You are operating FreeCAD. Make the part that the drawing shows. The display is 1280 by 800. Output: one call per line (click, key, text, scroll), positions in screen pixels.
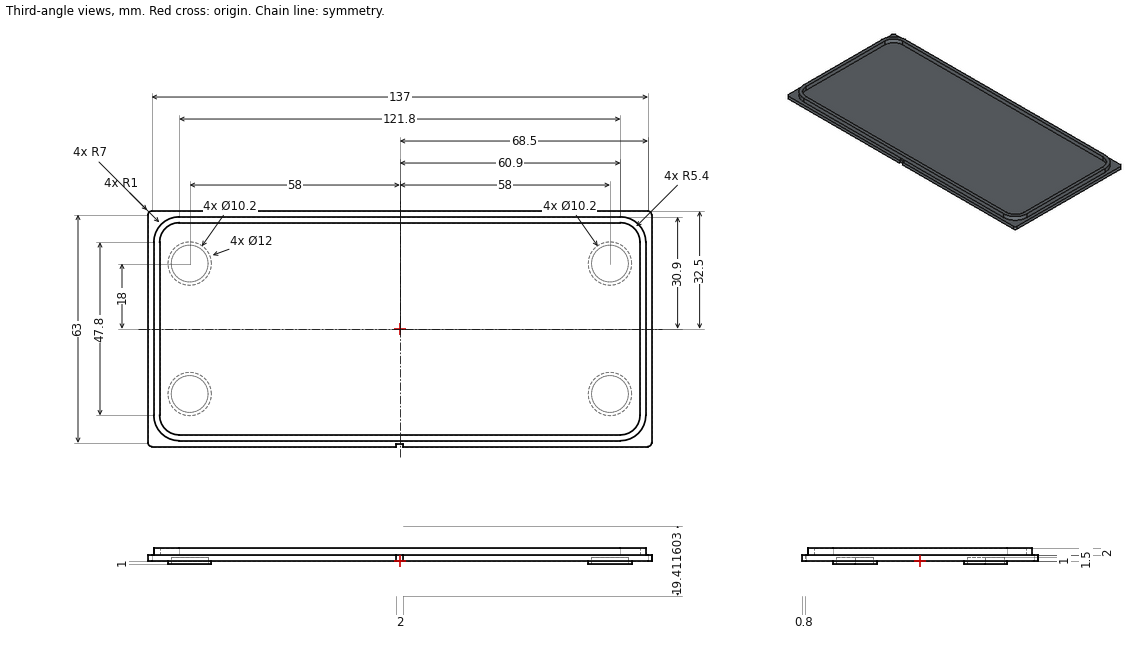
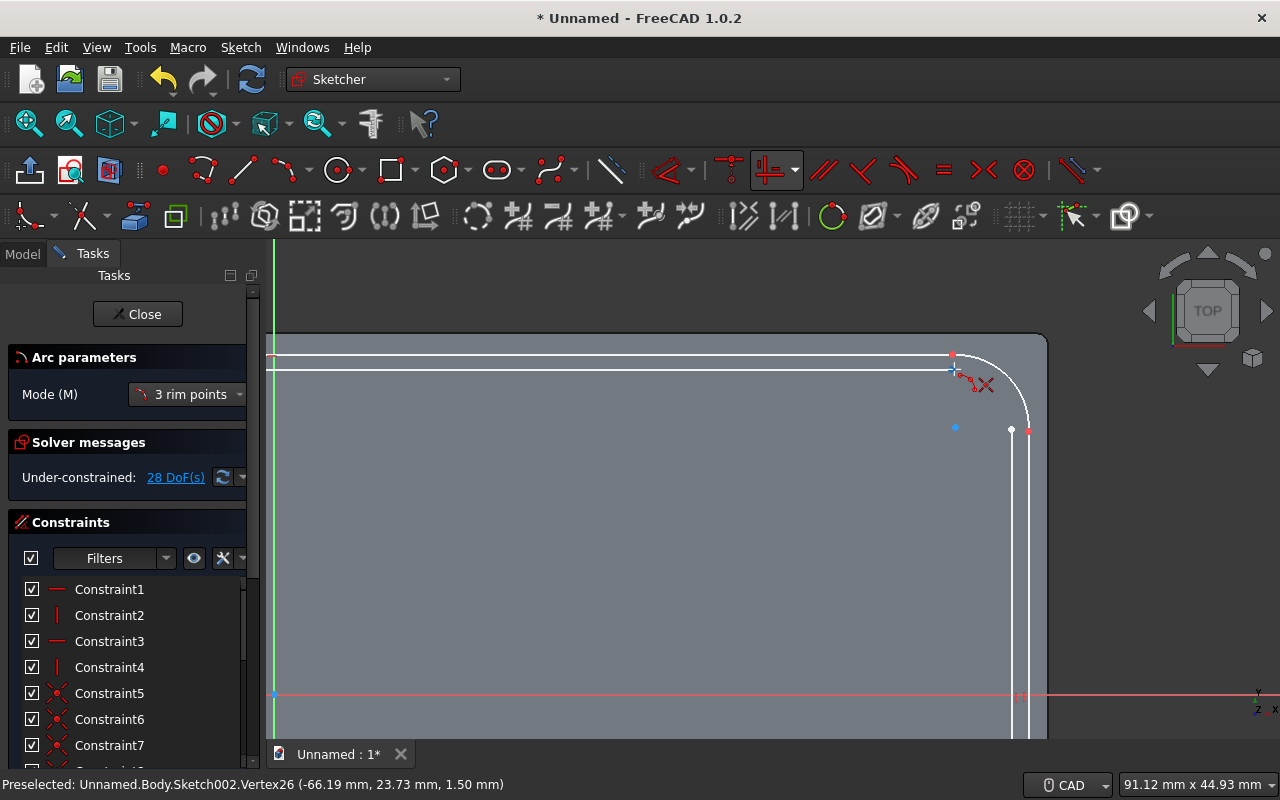
click(952, 370)
click(1012, 430)
click(995, 387)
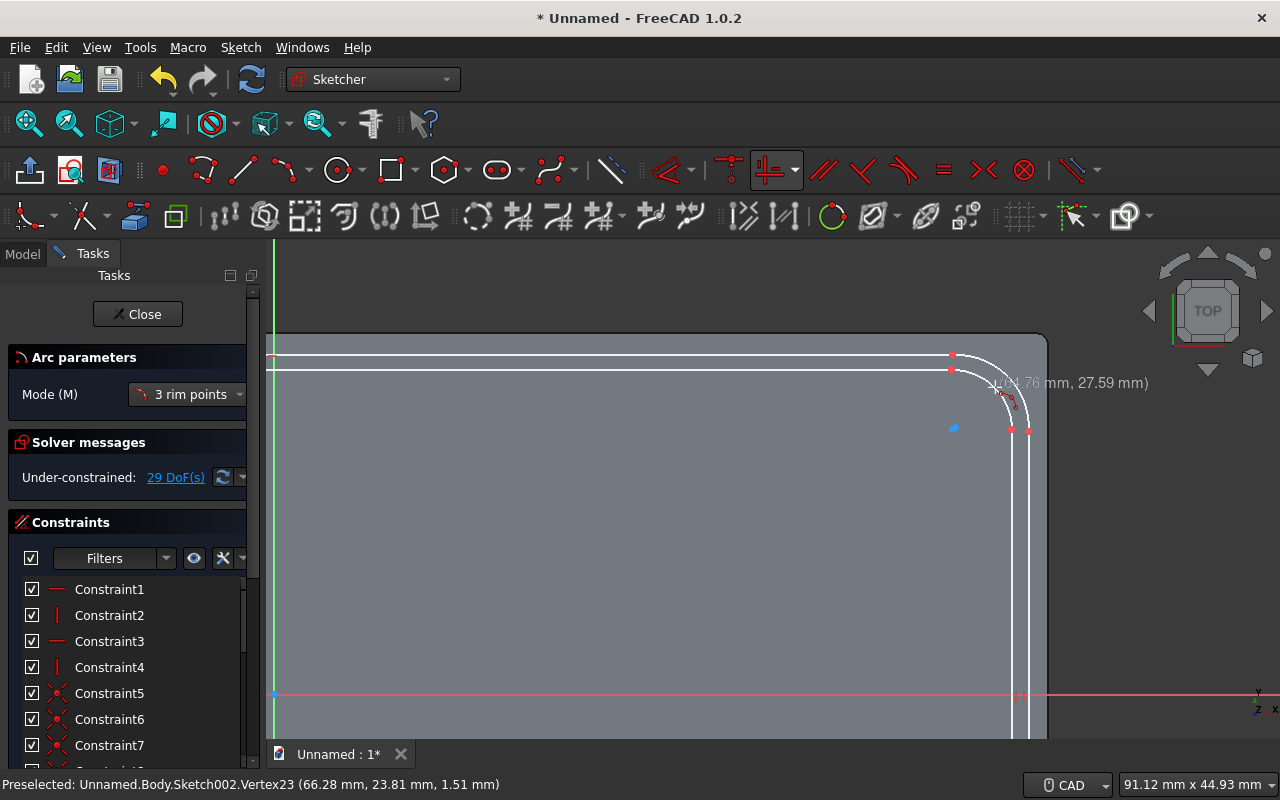
scroll(955, 369, down, 5)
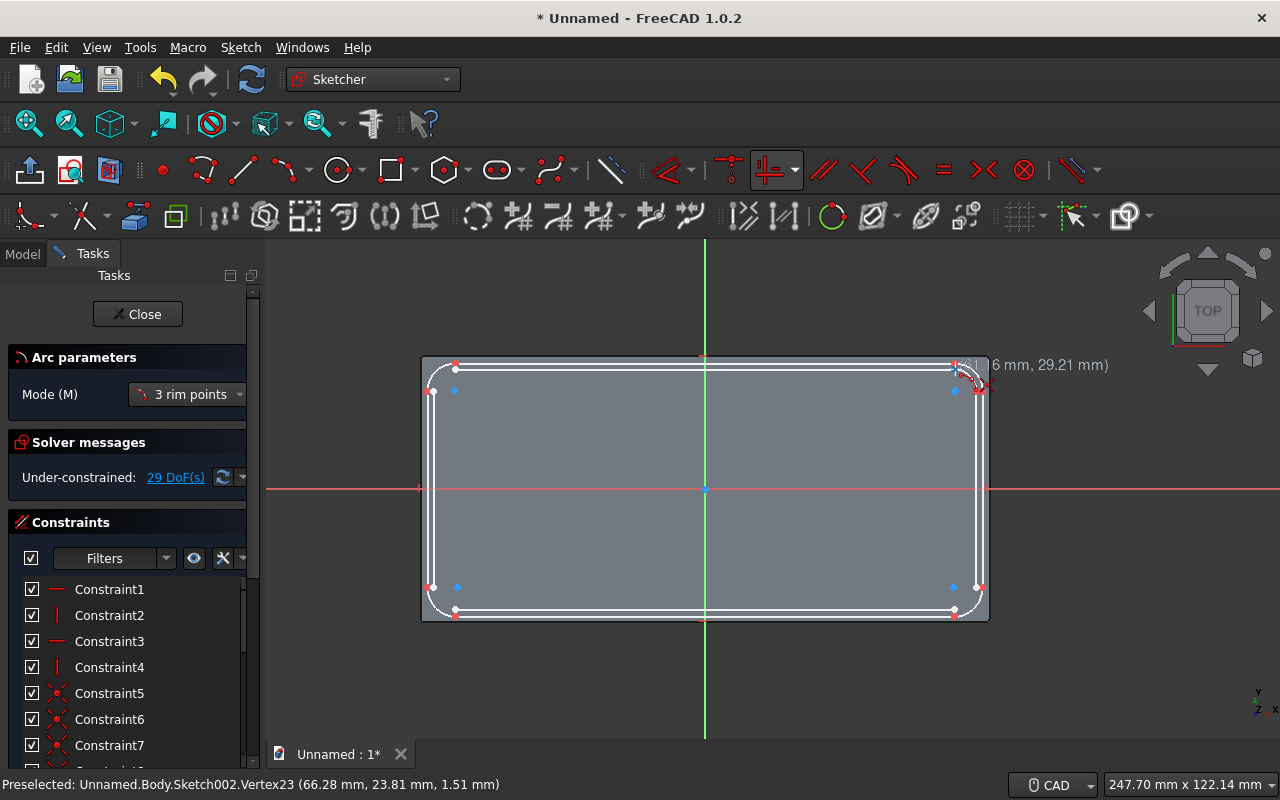
scroll(976, 587, up, 5)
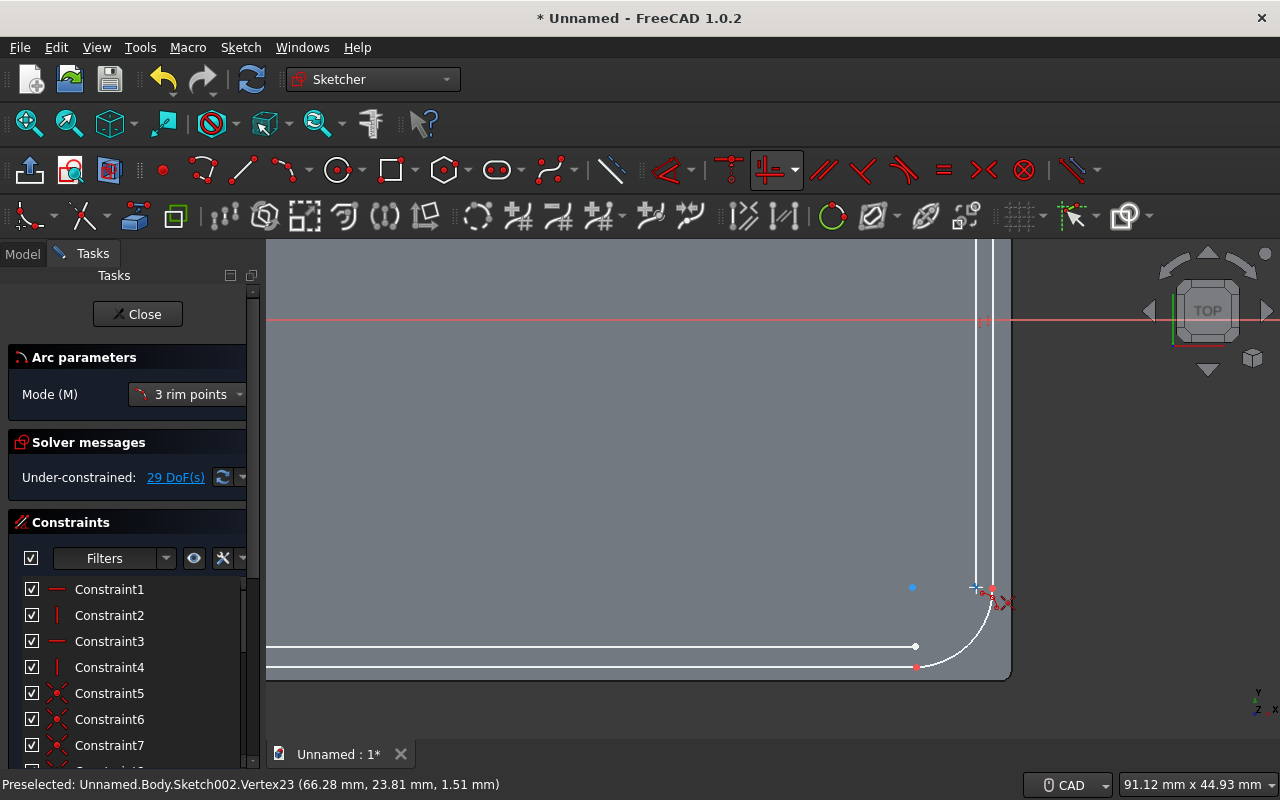
click(976, 587)
click(916, 647)
click(958, 628)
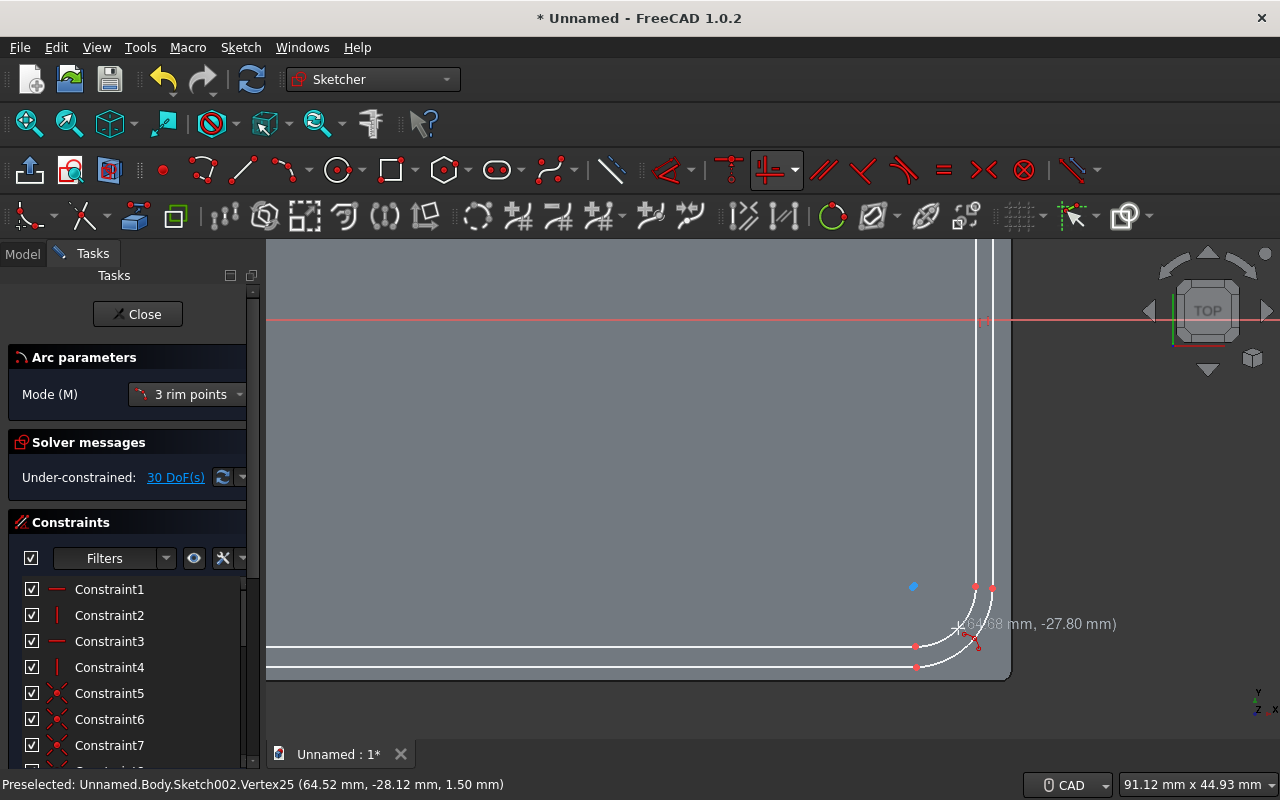
scroll(976, 588, down, 5)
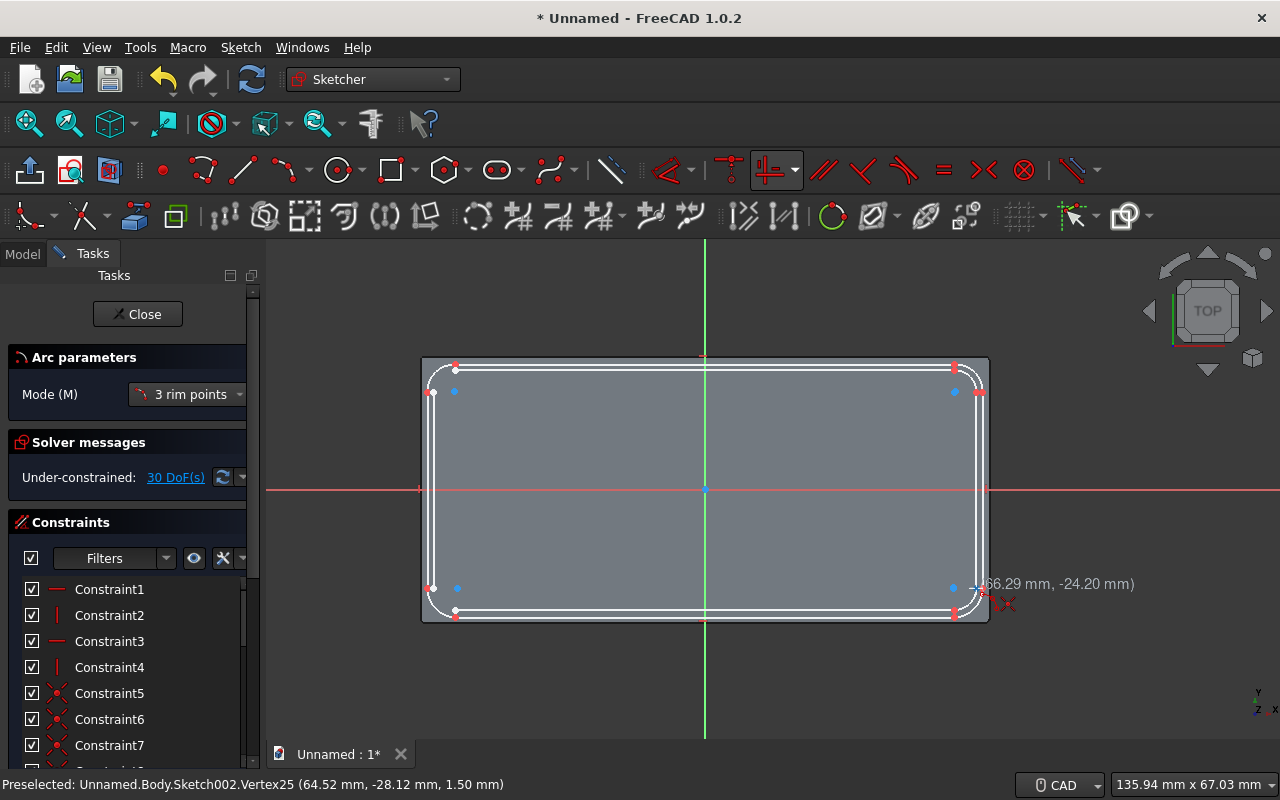
scroll(456, 610, up, 5)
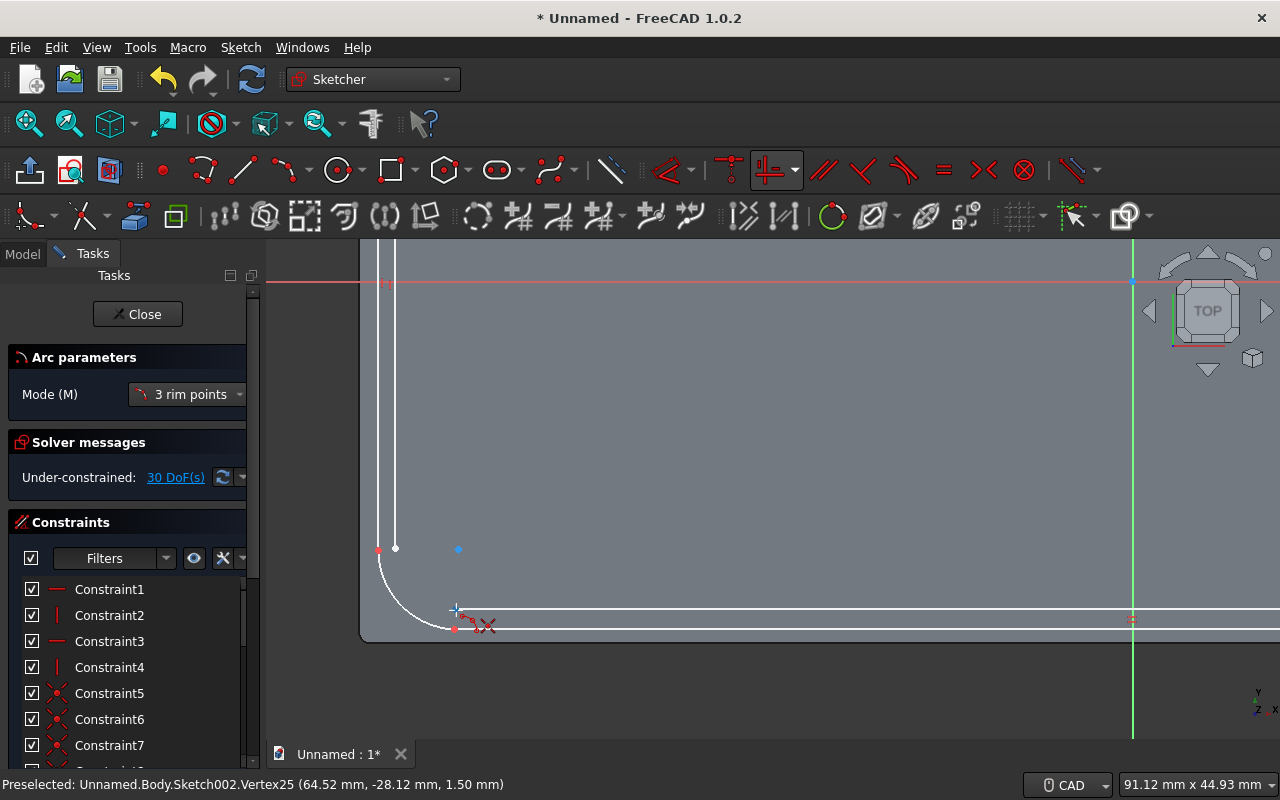
click(455, 609)
click(395, 549)
click(413, 590)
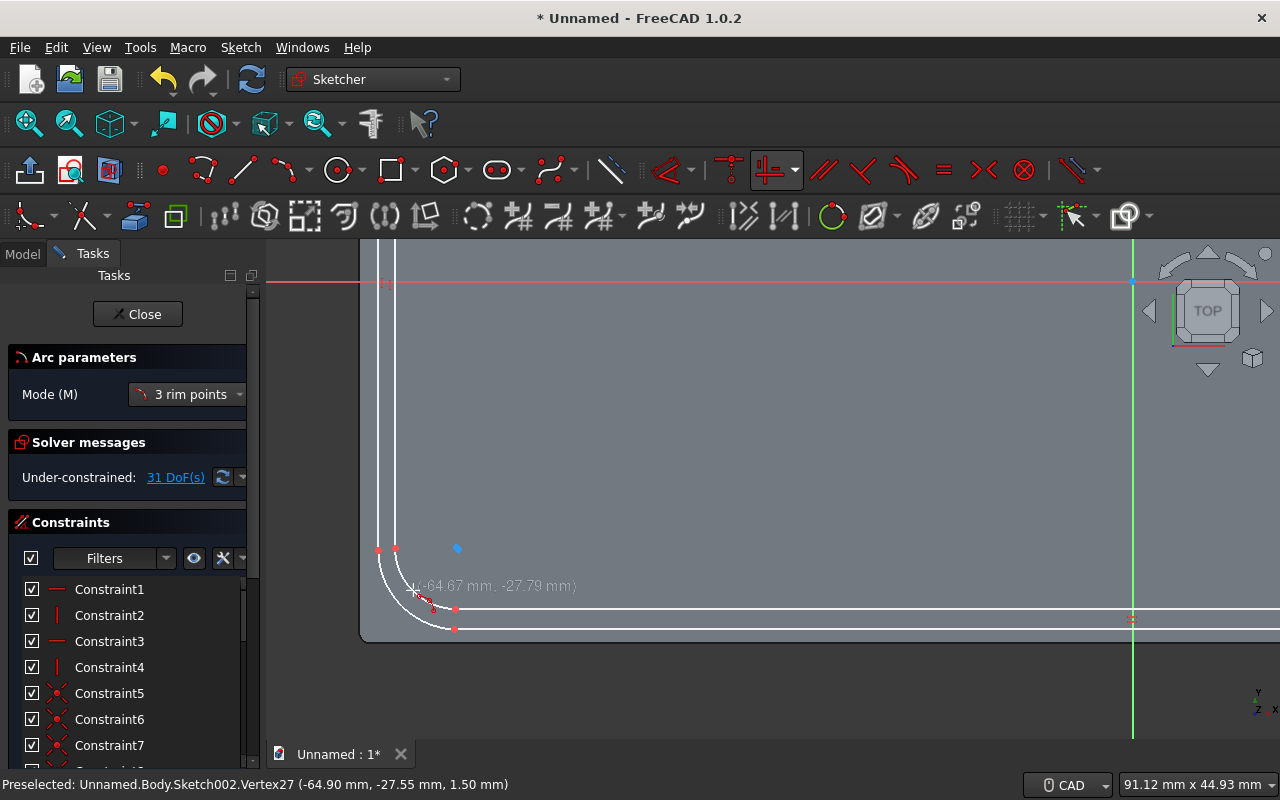
scroll(455, 610, down, 5)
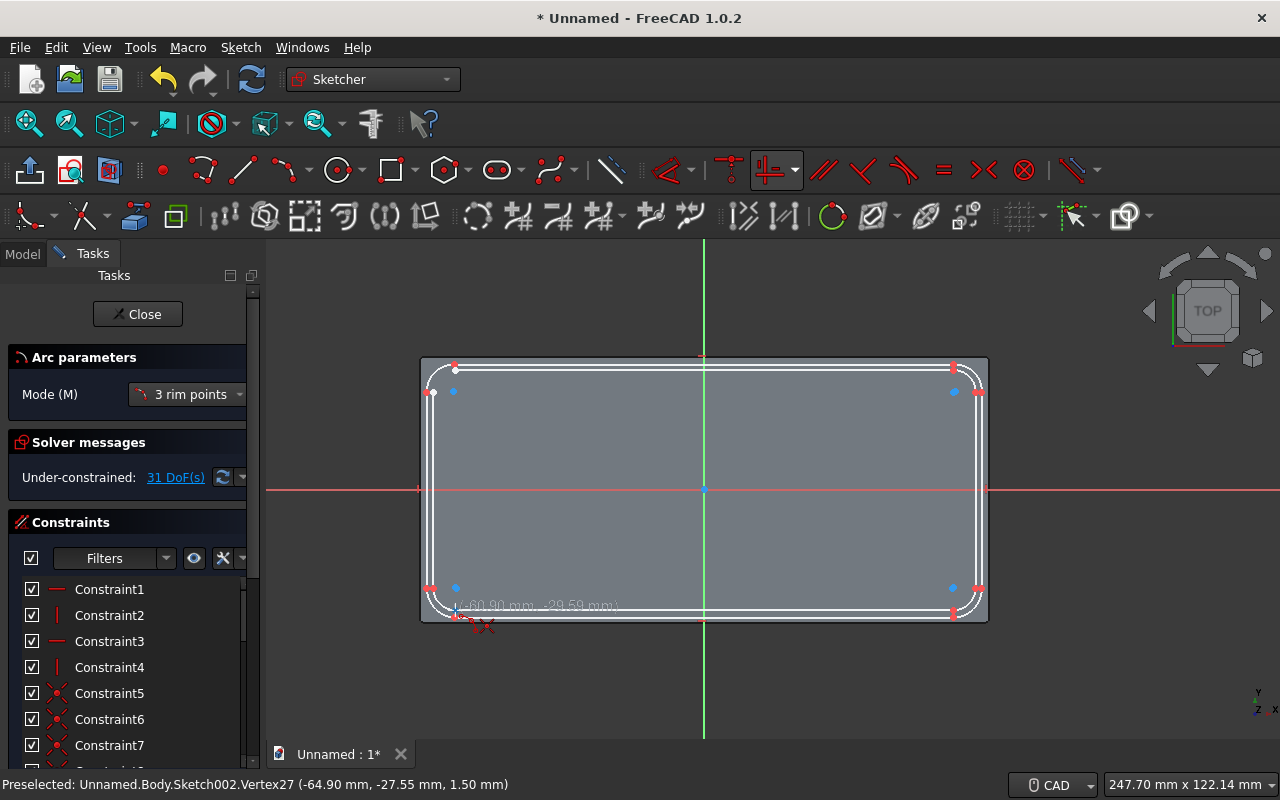
scroll(433, 392, up, 5)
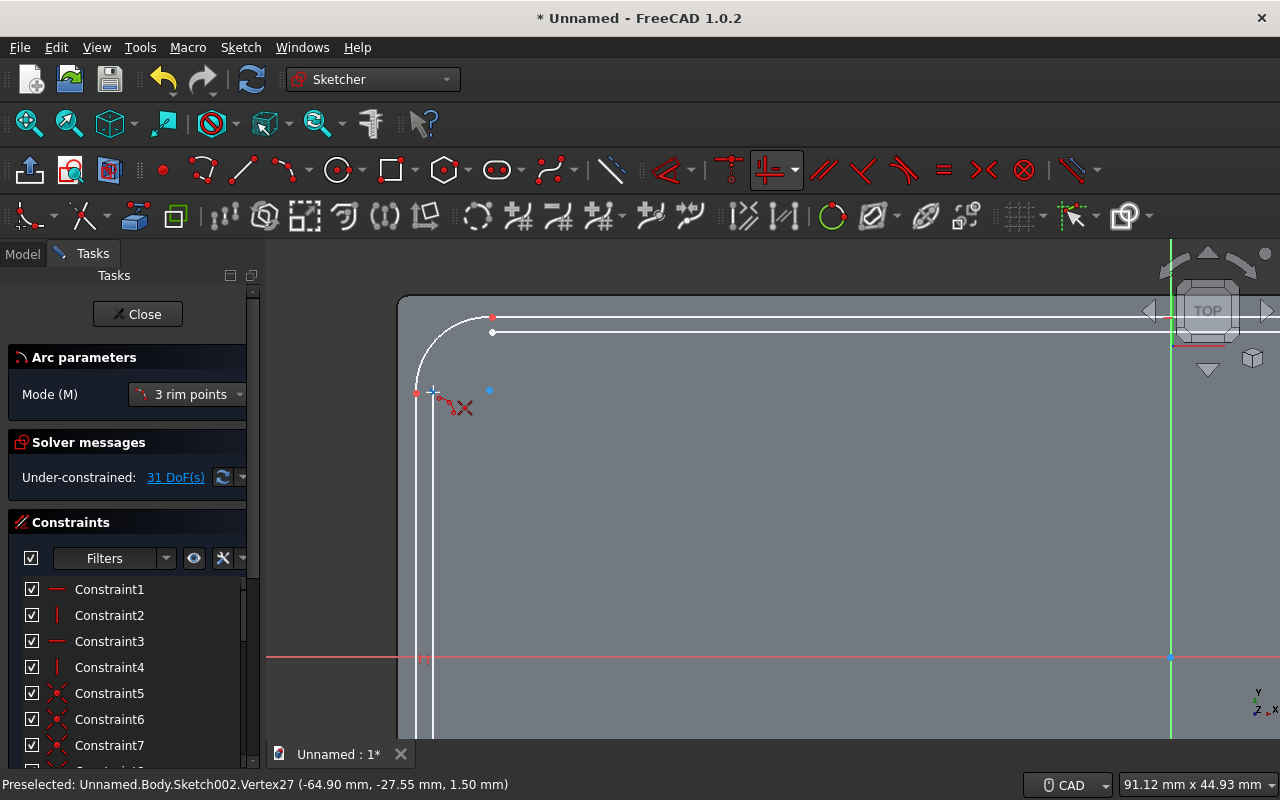
click(433, 392)
click(493, 332)
click(450, 349)
key(Escape)